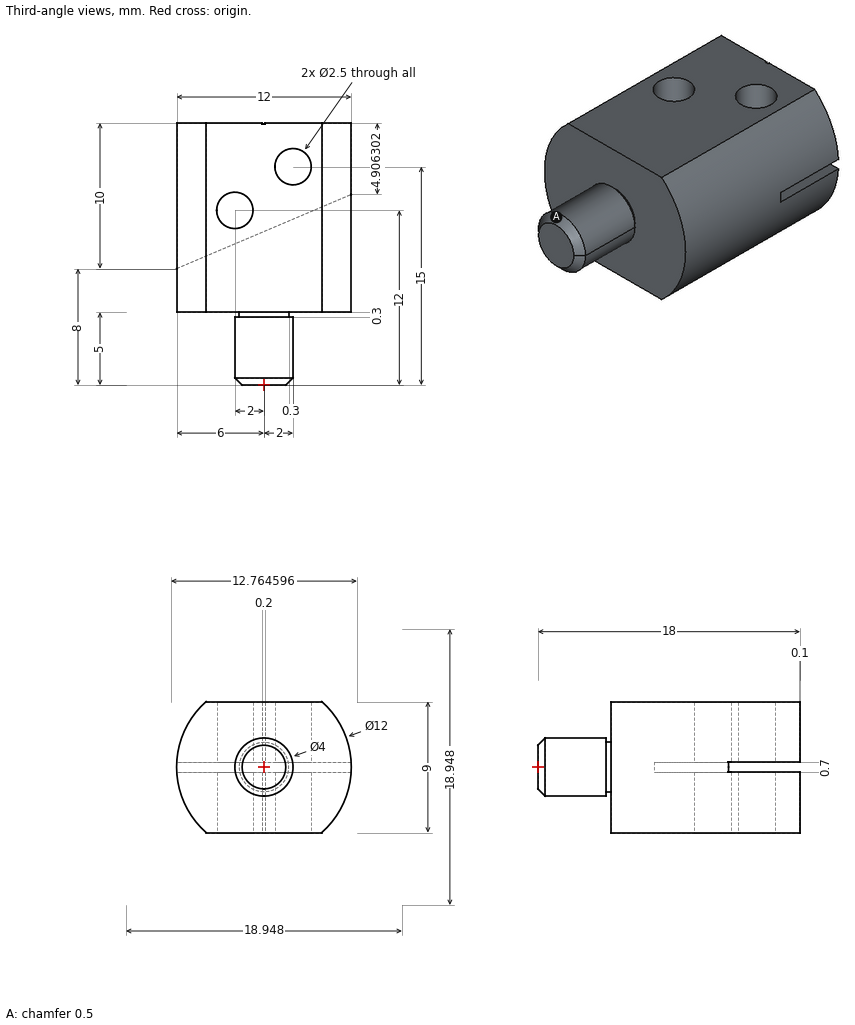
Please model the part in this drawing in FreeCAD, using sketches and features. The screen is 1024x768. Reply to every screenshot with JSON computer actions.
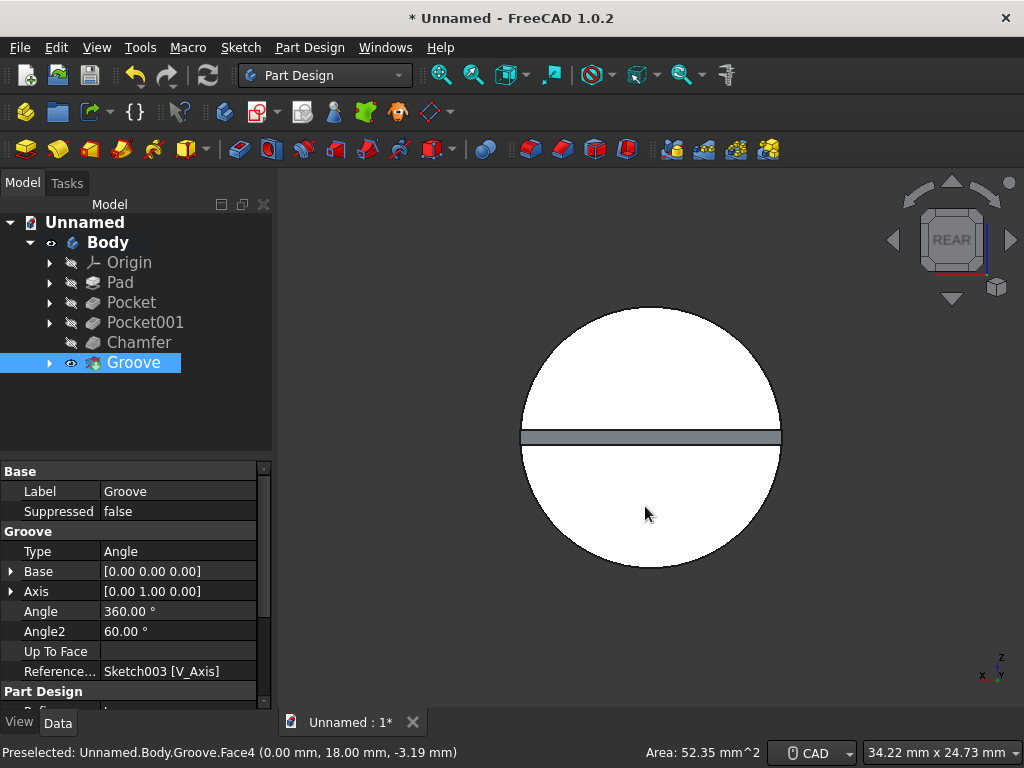
{"action": "left_click", "coordinate": [258, 112]}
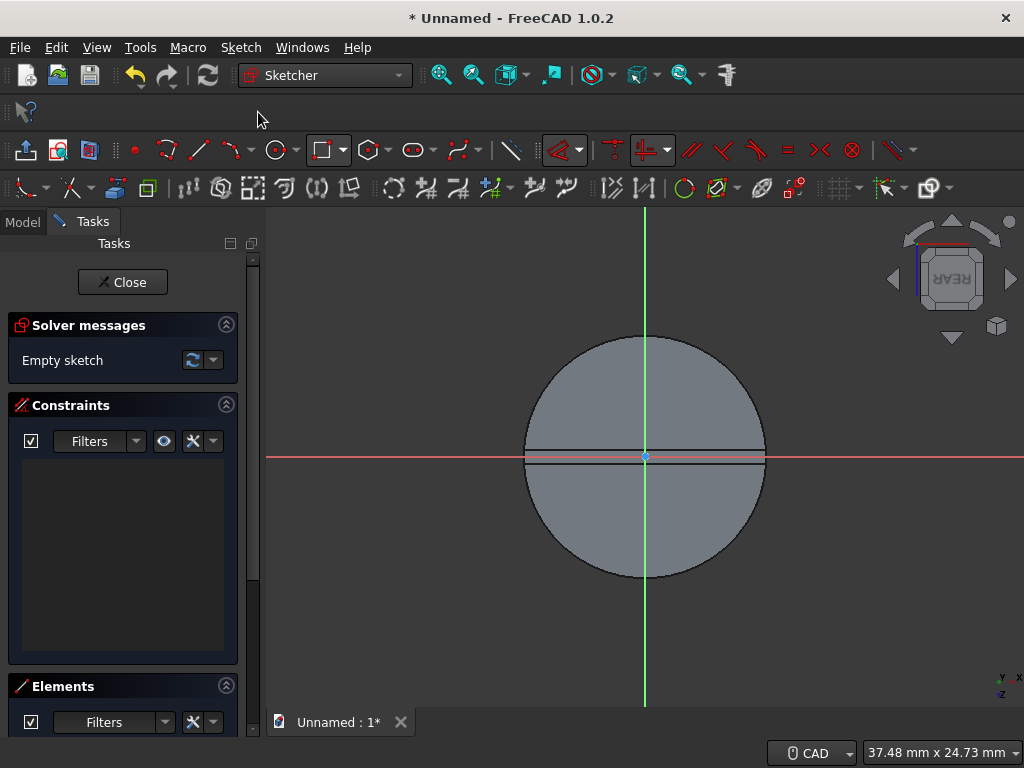
{"action": "scroll", "coordinate": [294, 457], "scroll_direction": "down", "scroll_amount": 1}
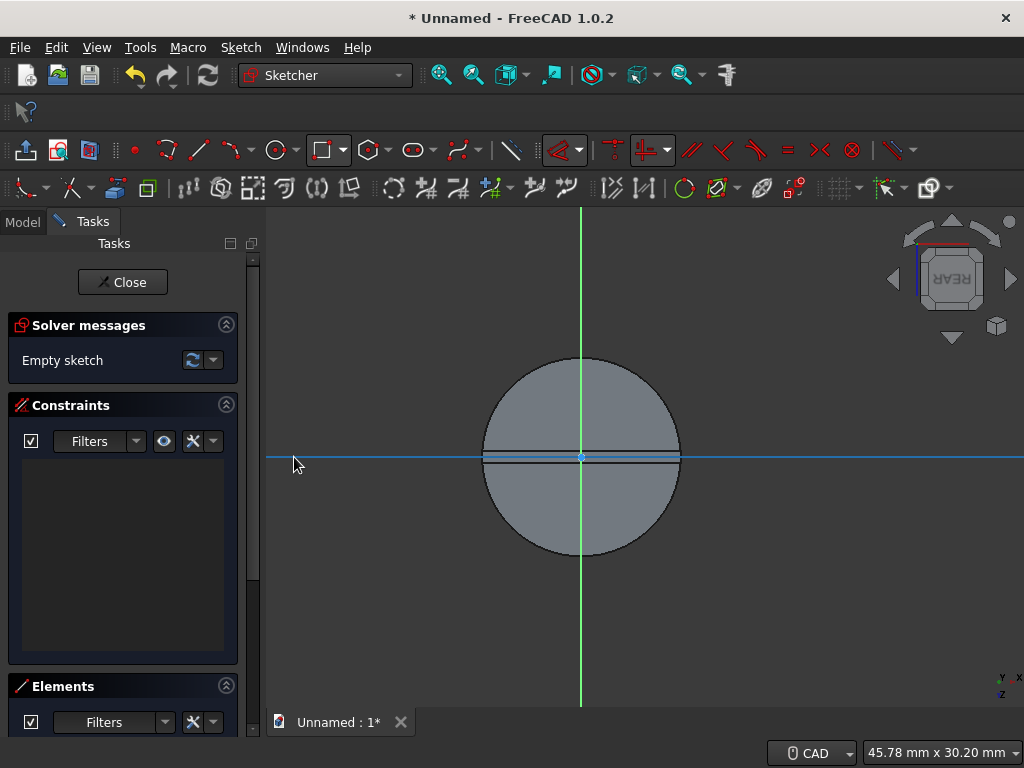
{"action": "key", "text": "g v"}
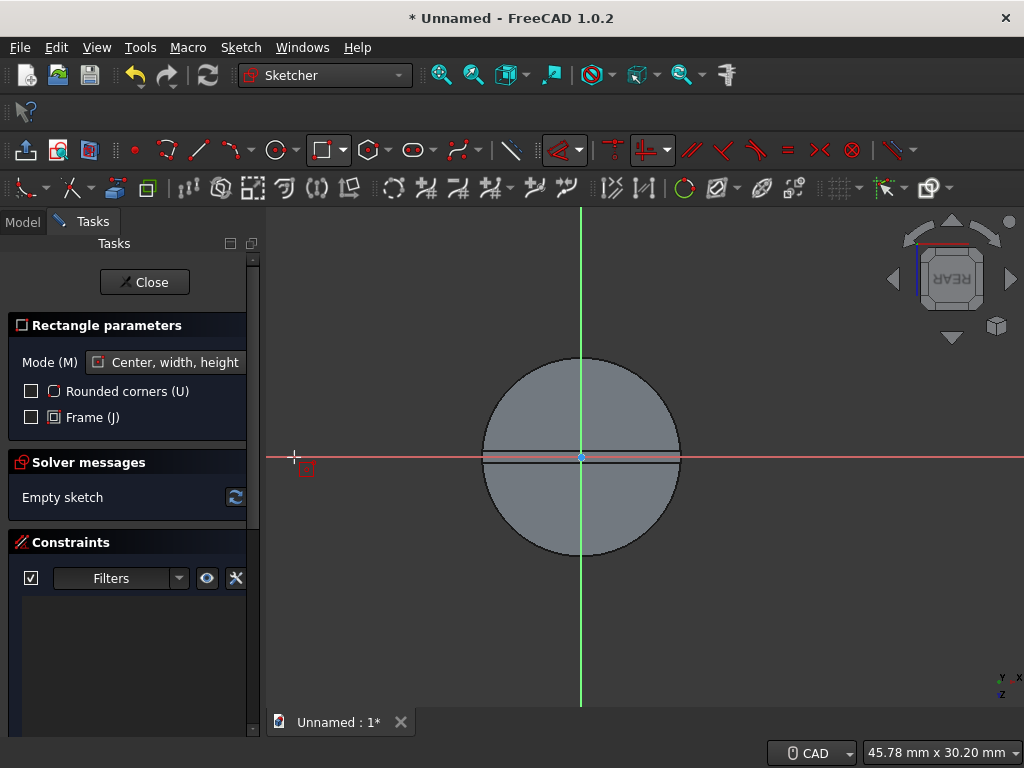
{"action": "left_click", "coordinate": [581, 457]}
{"action": "left_click", "coordinate": [738, 300]}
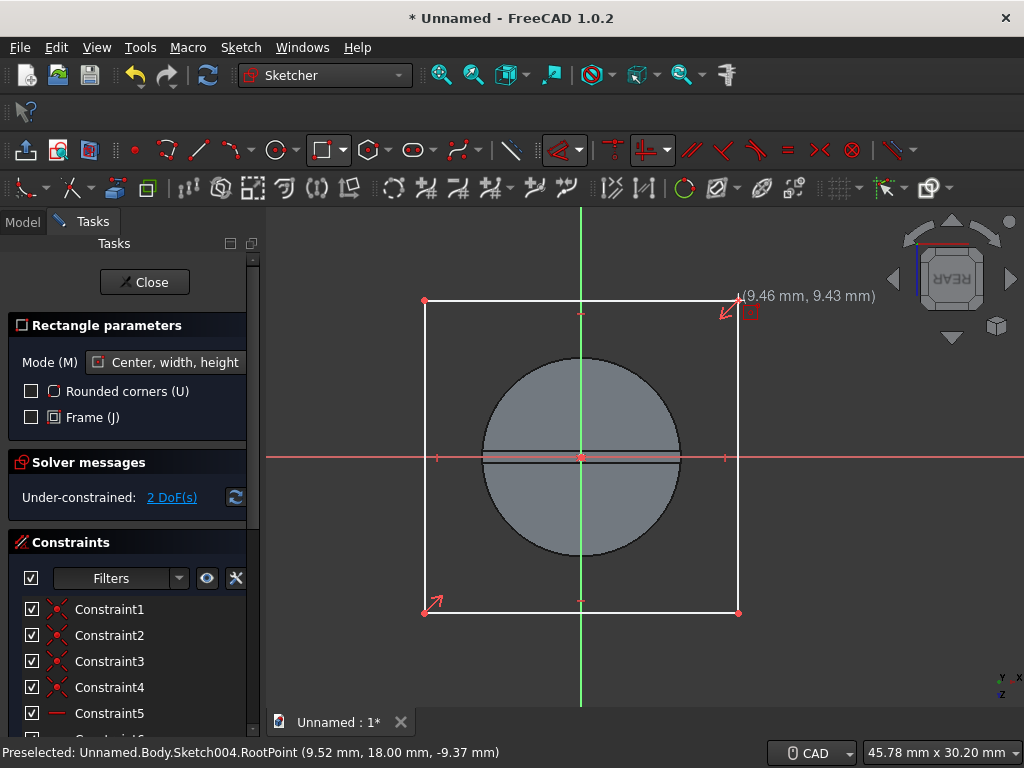
{"action": "left_click", "coordinate": [581, 457]}
{"action": "left_click", "coordinate": [687, 383]}
{"action": "key", "text": "Escape"}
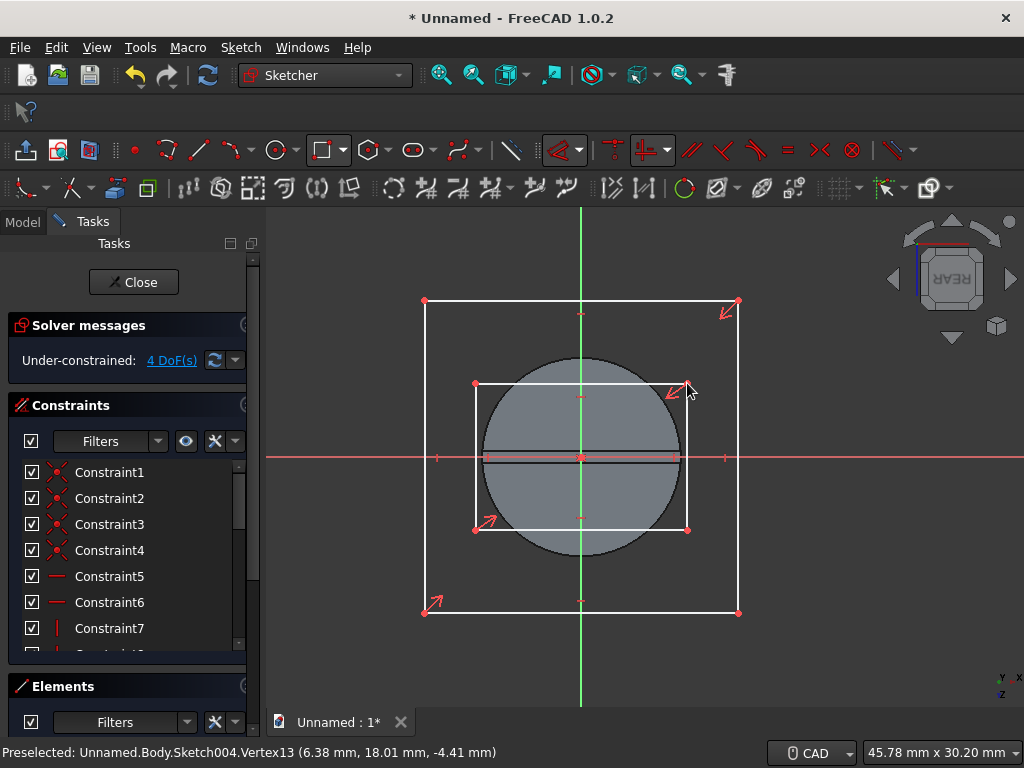
{"action": "left_click", "coordinate": [687, 486]}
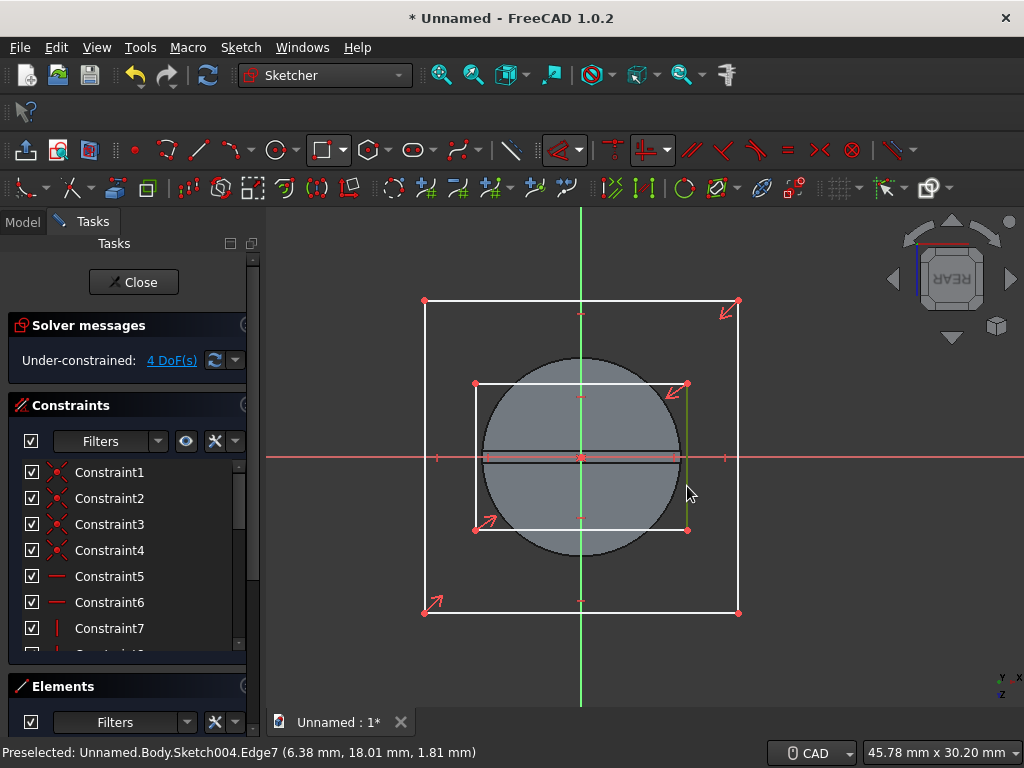
{"action": "key", "text": "i"}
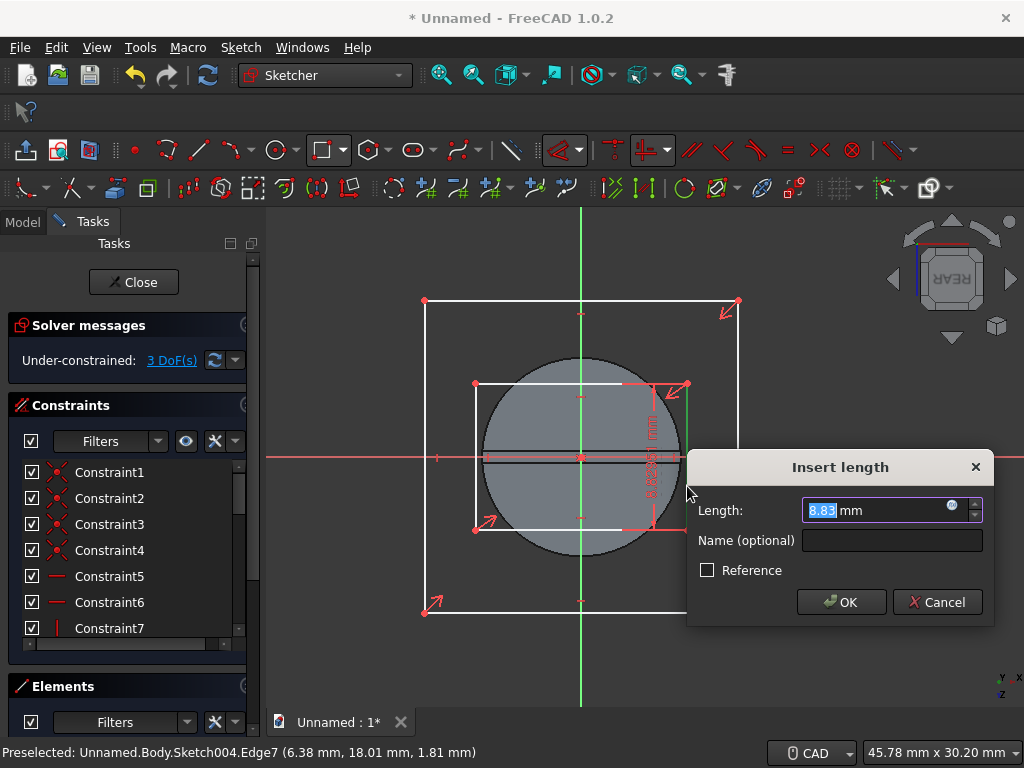
{"action": "type", "text": "9"}
{"action": "key", "text": "Return"}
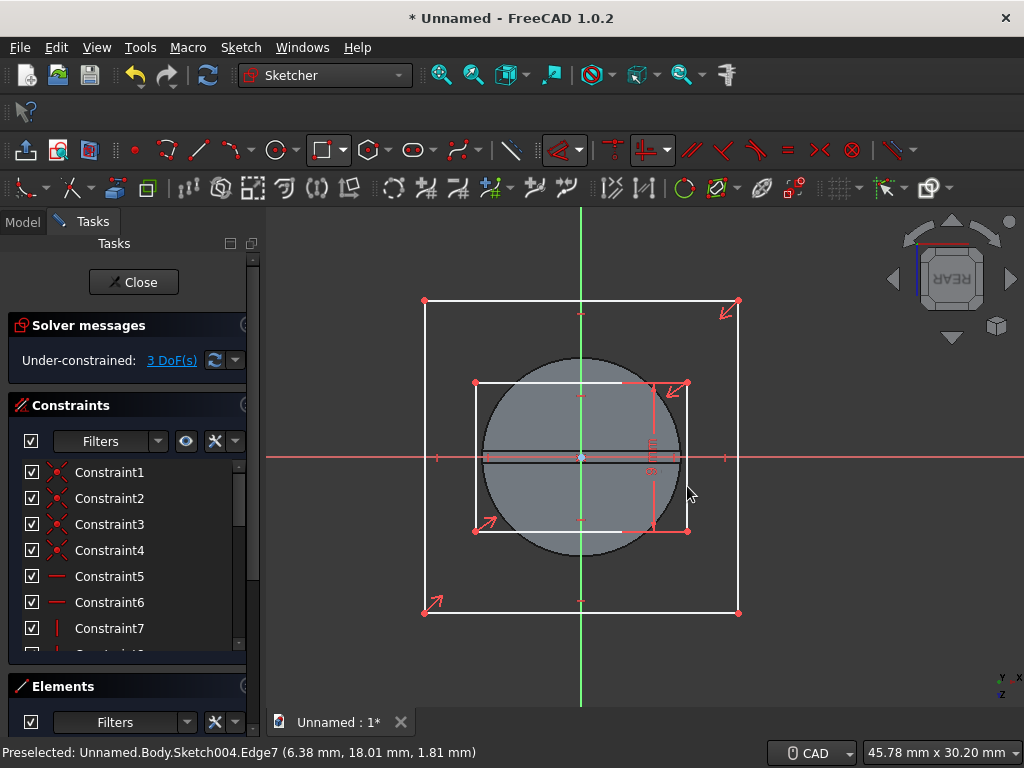
{"action": "left_click", "coordinate": [519, 613]}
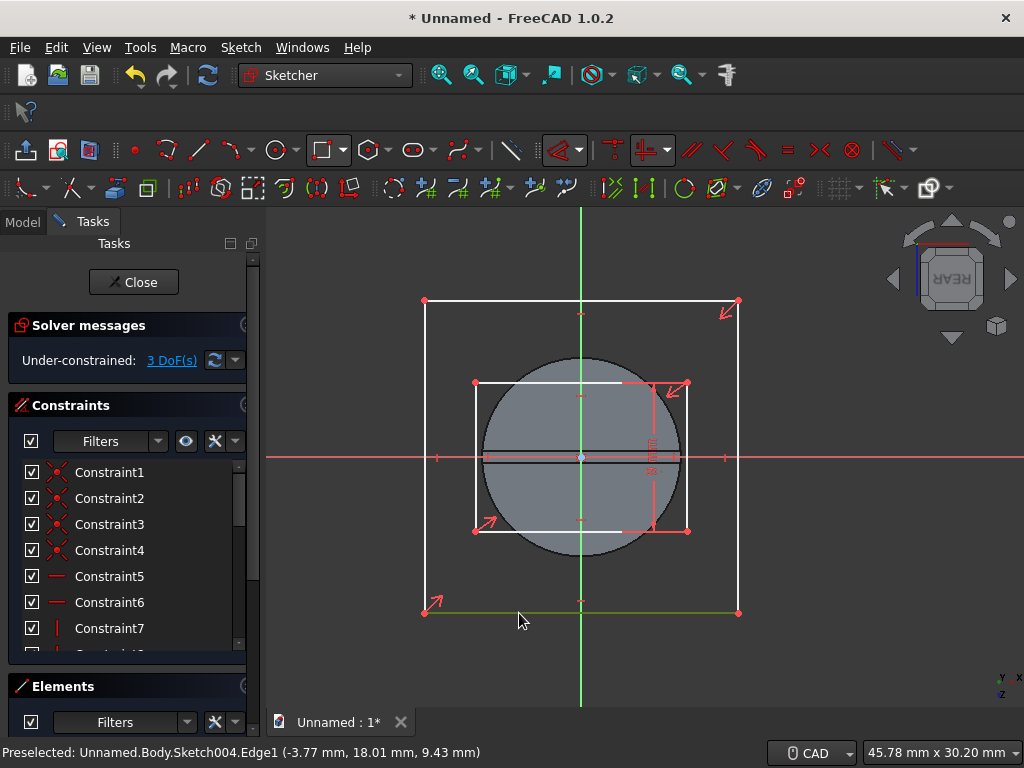
{"action": "key", "text": "l"}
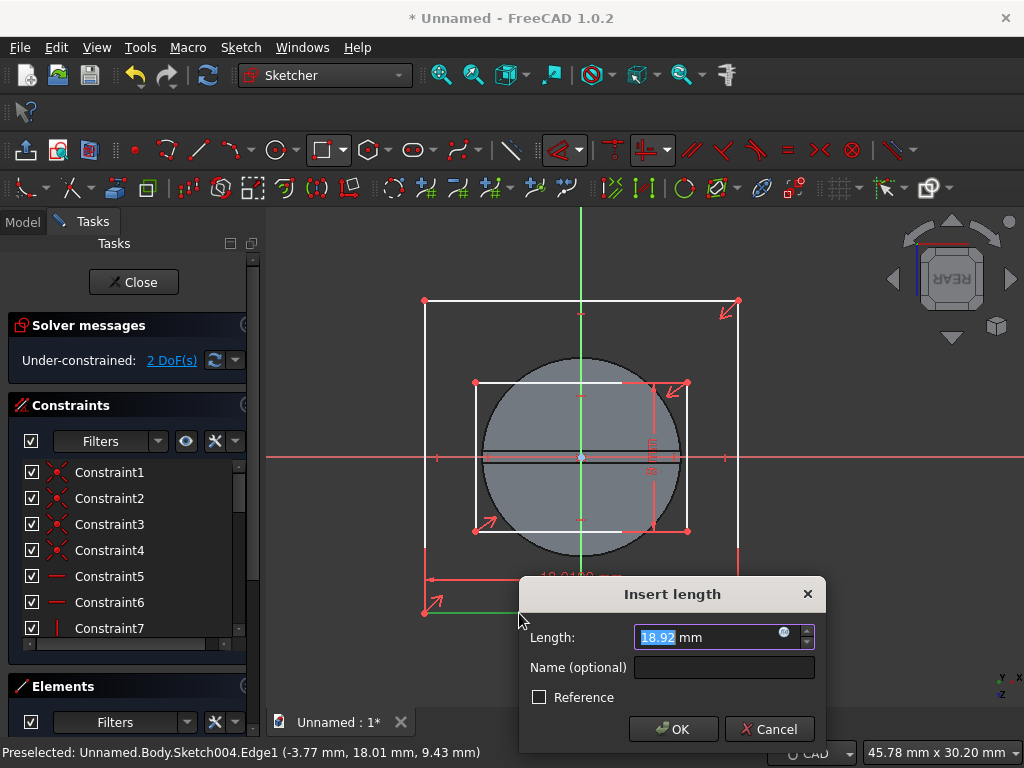
{"action": "type", "text": "18.948"}
{"action": "key", "text": "Return"}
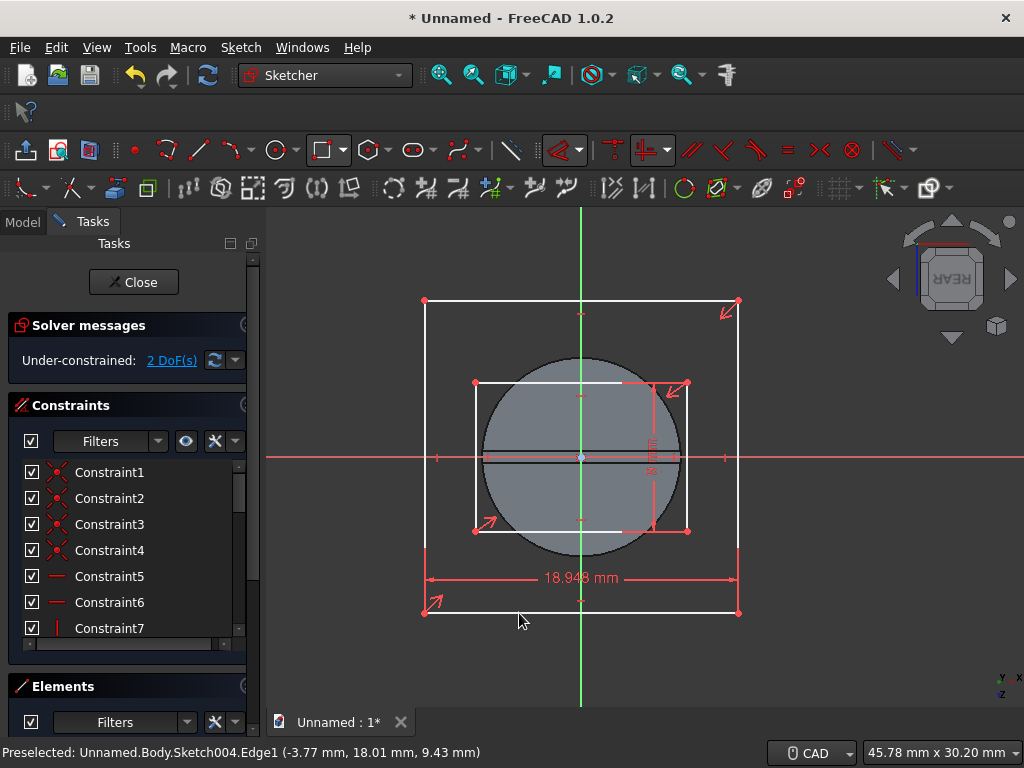
{"action": "left_click", "coordinate": [738, 520]}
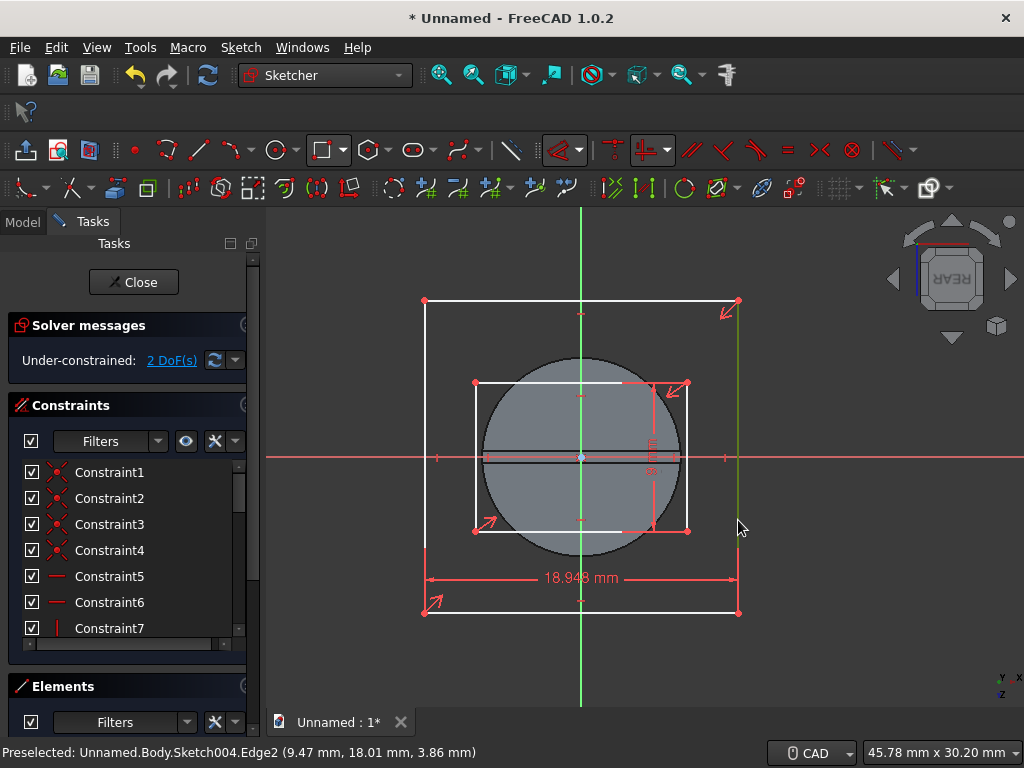
{"action": "key", "text": "i"}